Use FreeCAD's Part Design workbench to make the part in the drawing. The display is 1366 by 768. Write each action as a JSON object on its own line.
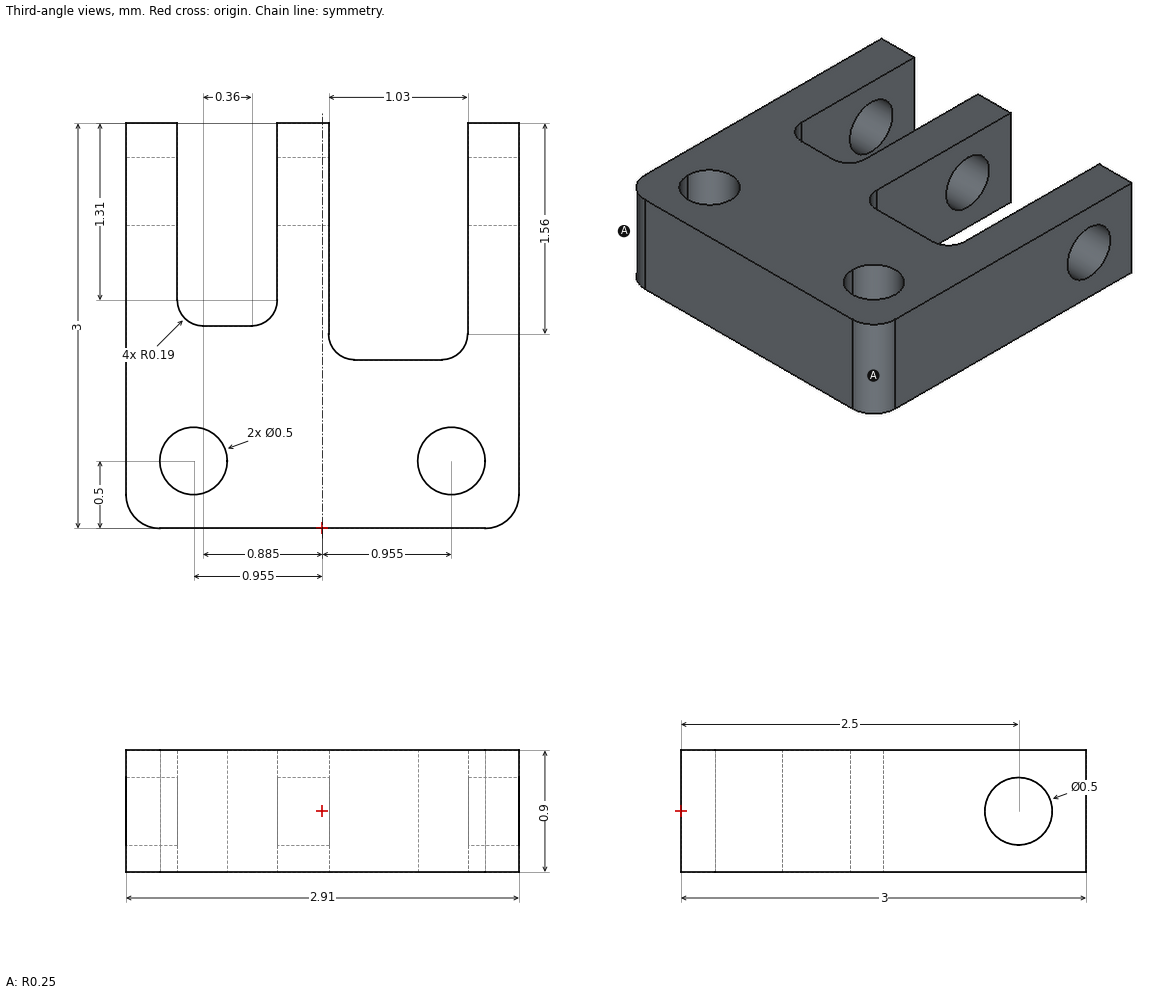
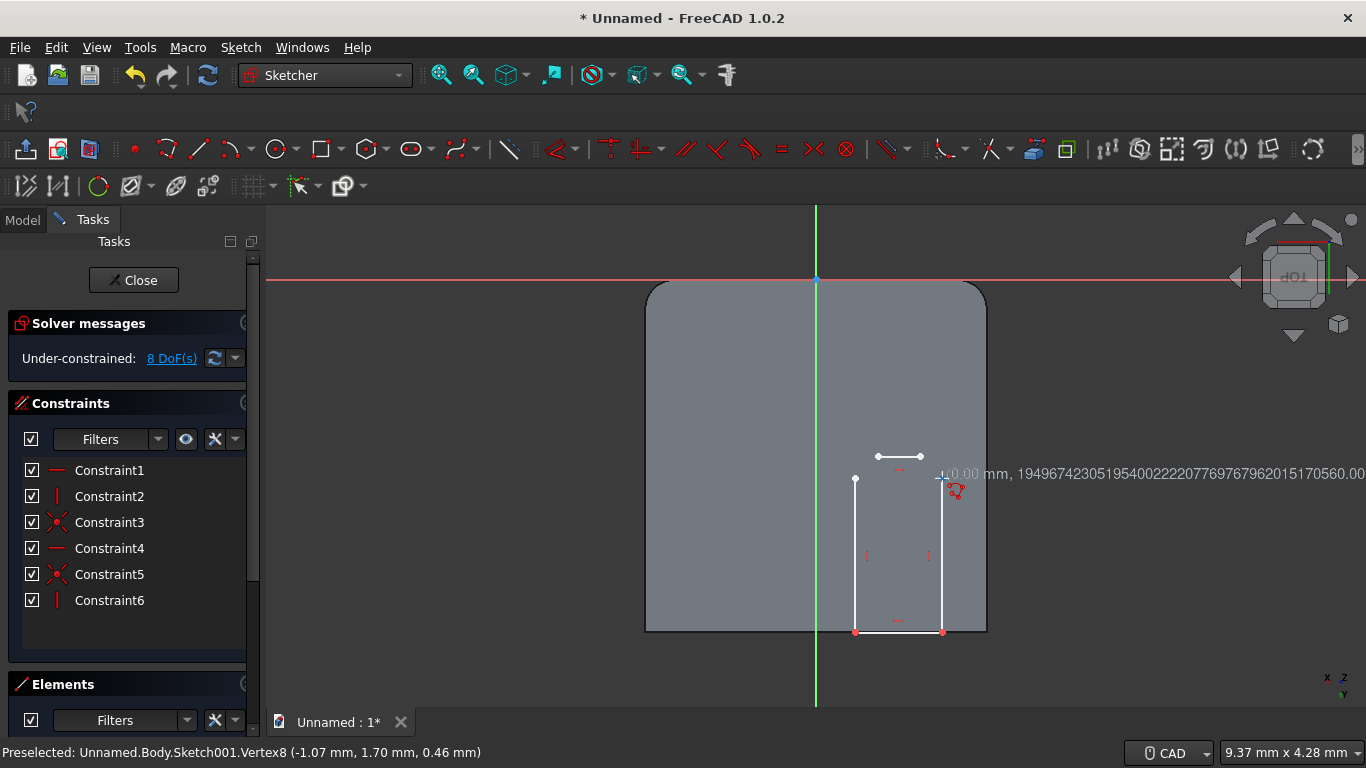
{"action": "key", "text": "g 3 a"}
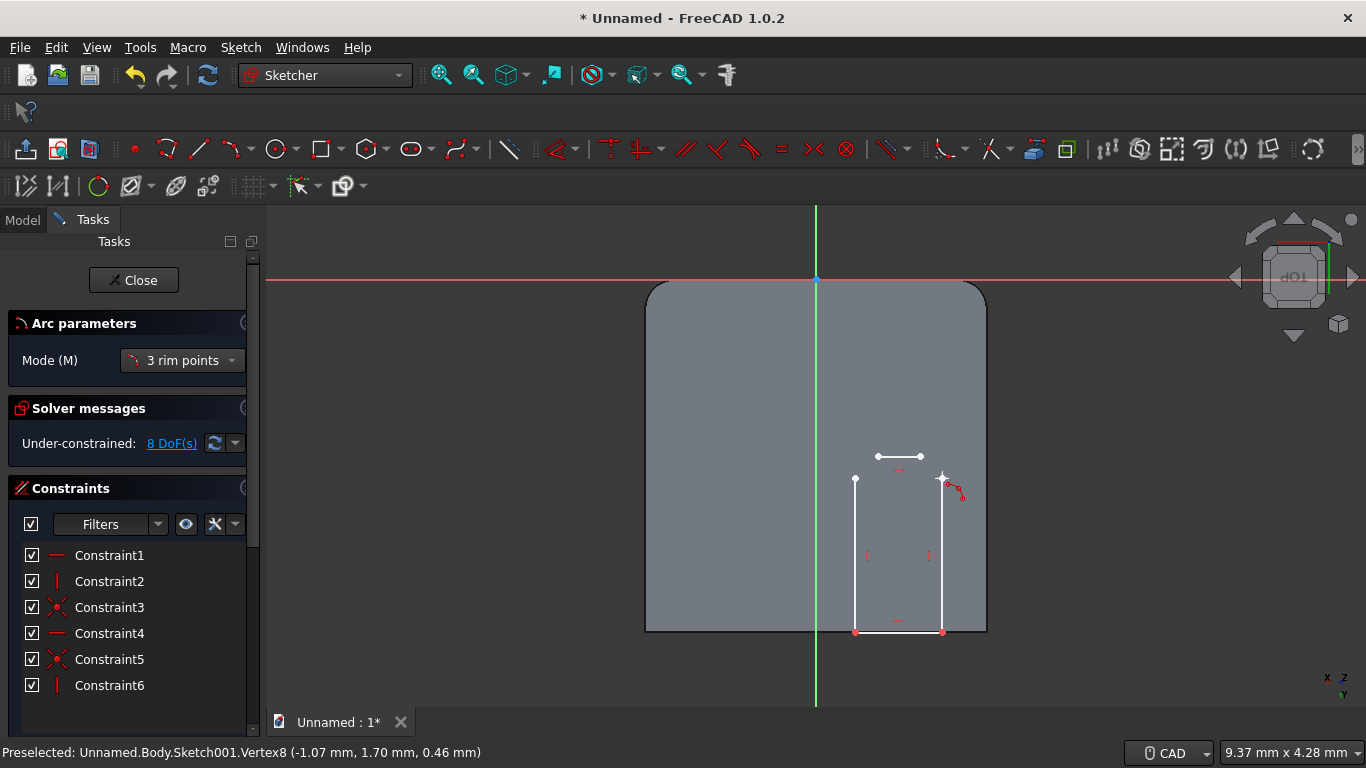
{"action": "left_click", "coordinate": [878, 457]}
{"action": "left_click", "coordinate": [855, 479]}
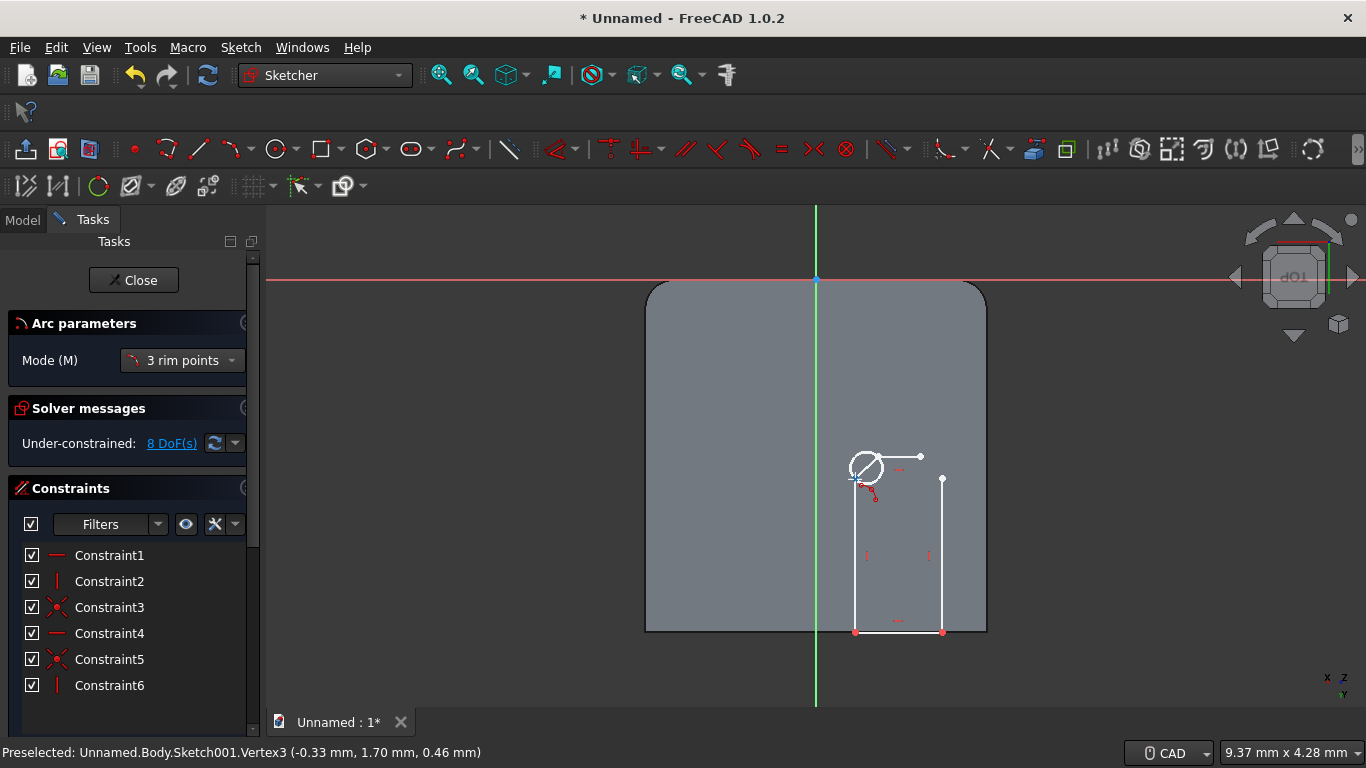
{"action": "scroll", "coordinate": [862, 463], "scroll_direction": "up", "scroll_amount": 5}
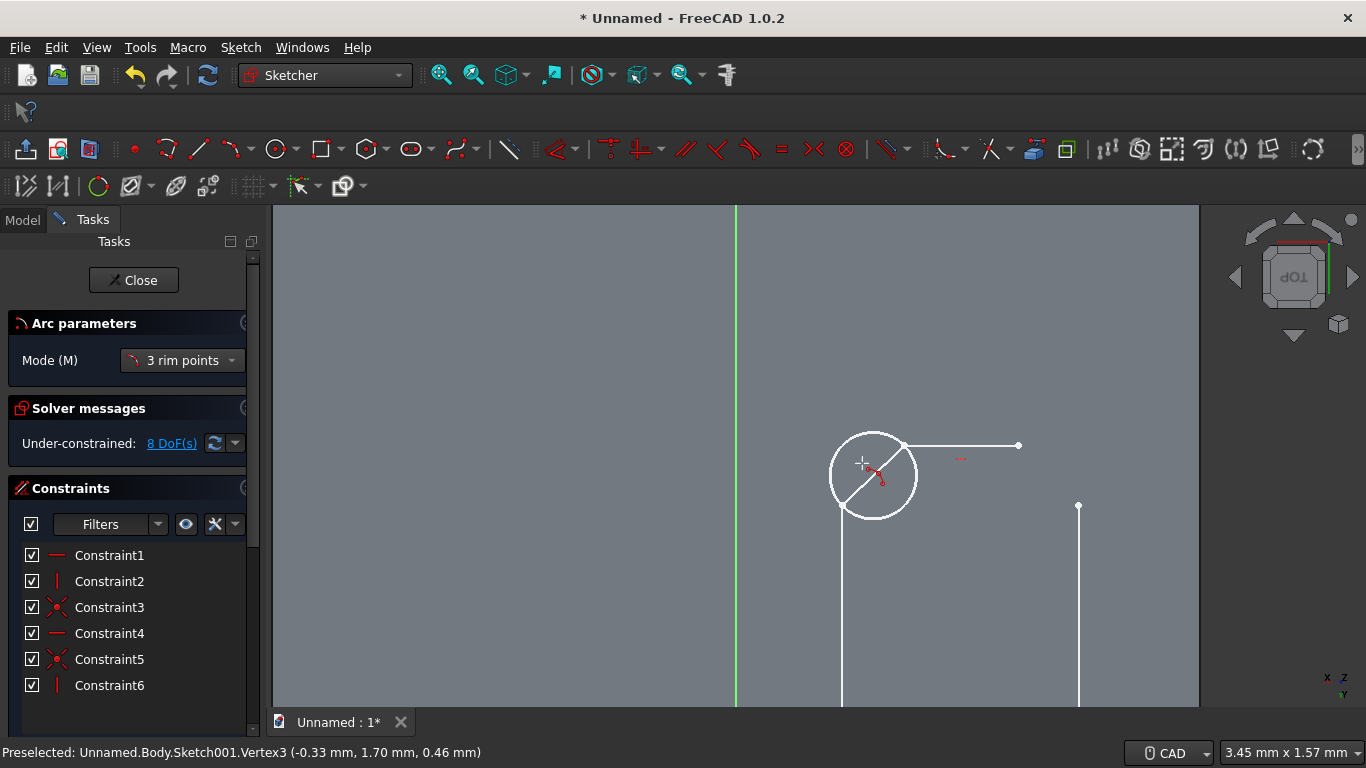
{"action": "left_click", "coordinate": [861, 461]}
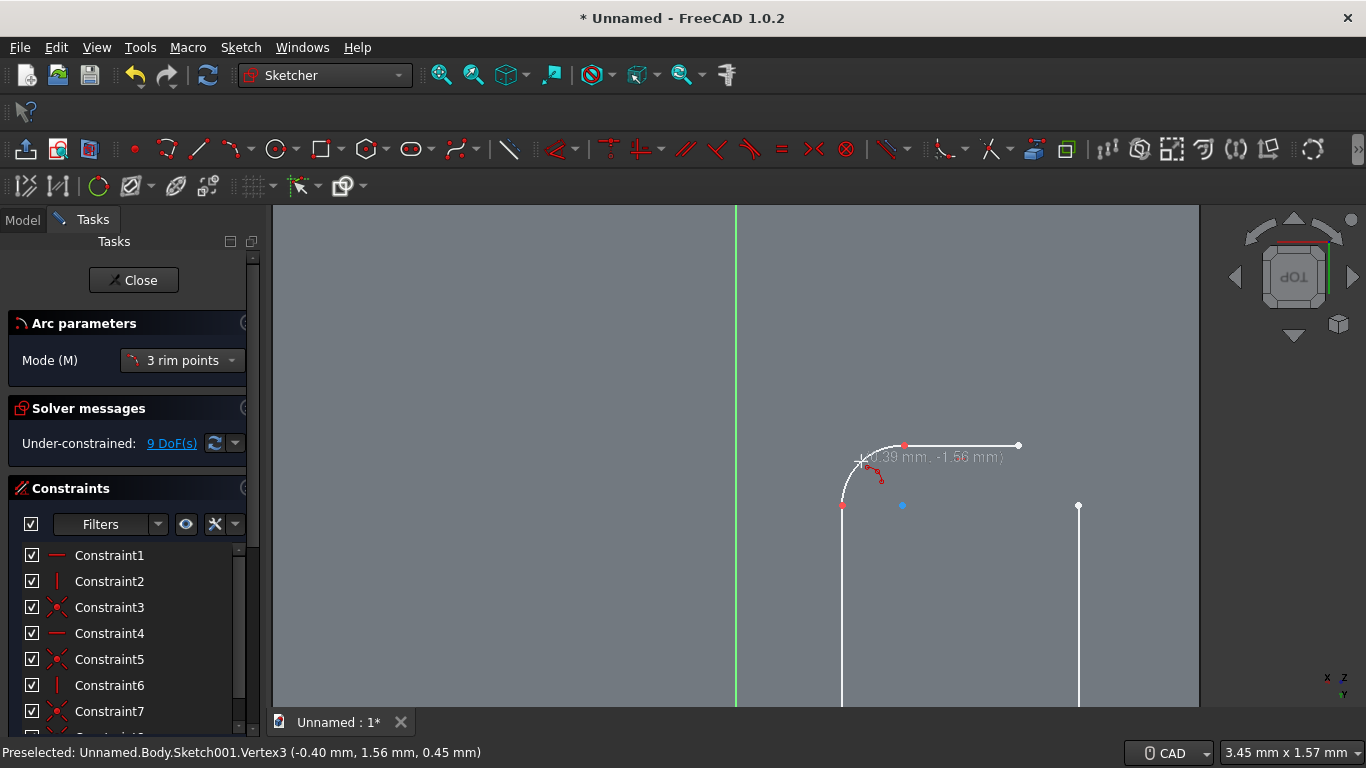
{"action": "left_click", "coordinate": [1079, 506]}
{"action": "left_click", "coordinate": [1019, 446]}
{"action": "left_click", "coordinate": [1061, 461]}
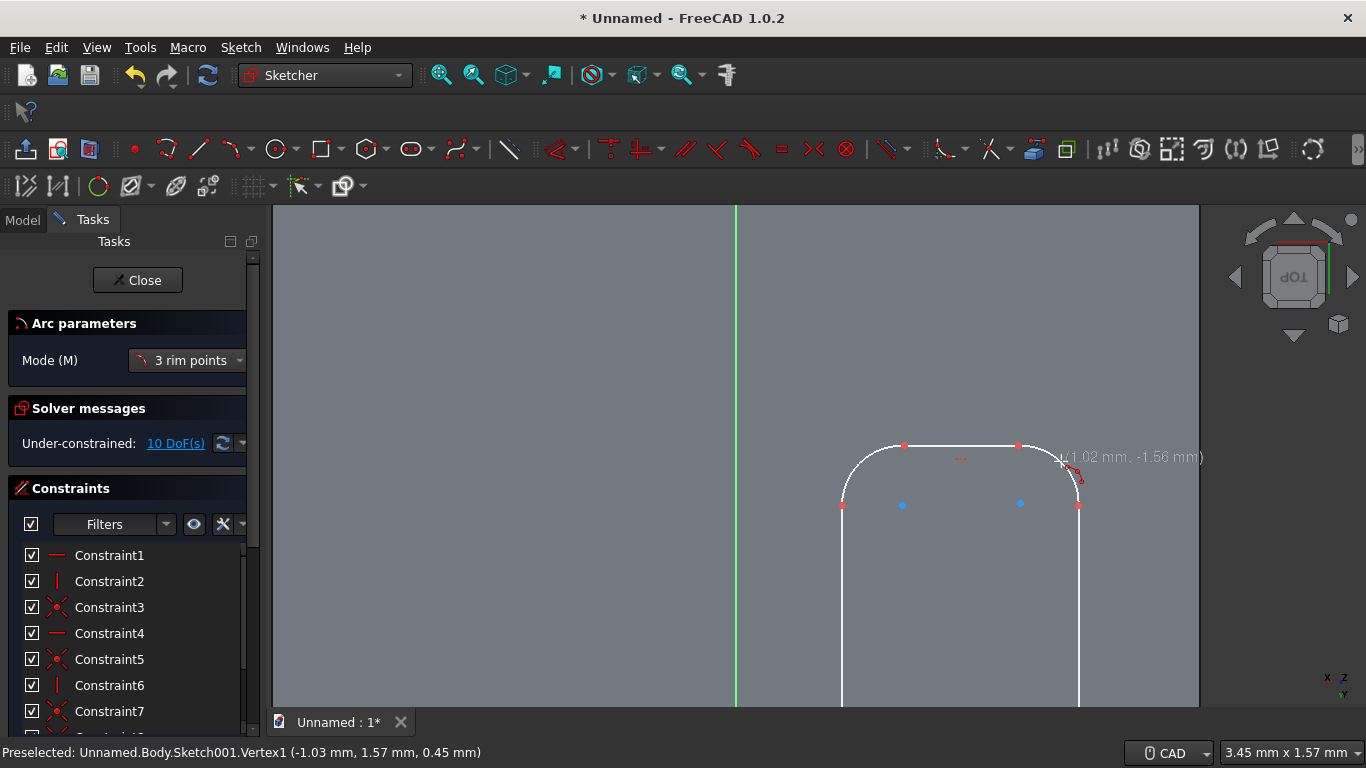
{"action": "left_click", "coordinate": [168, 150]}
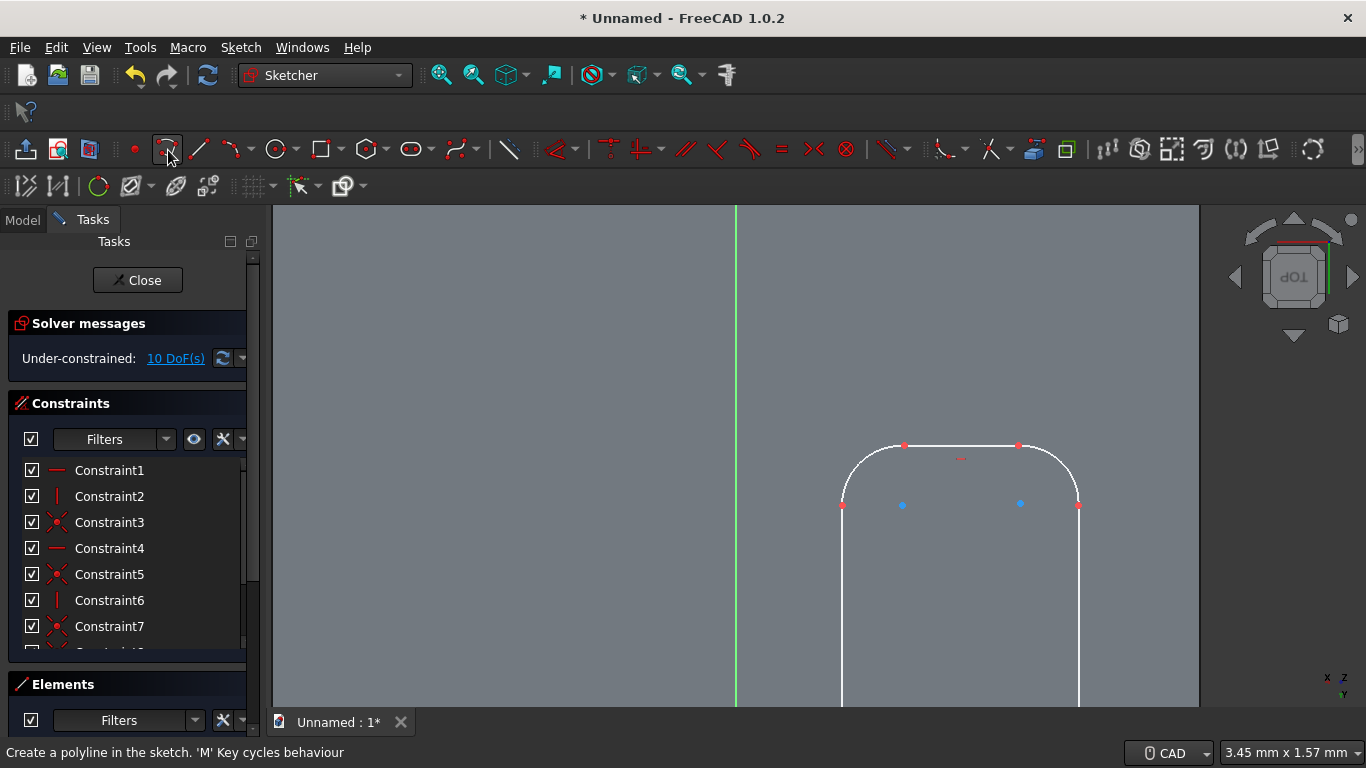
{"action": "left_click", "coordinate": [393, 424]}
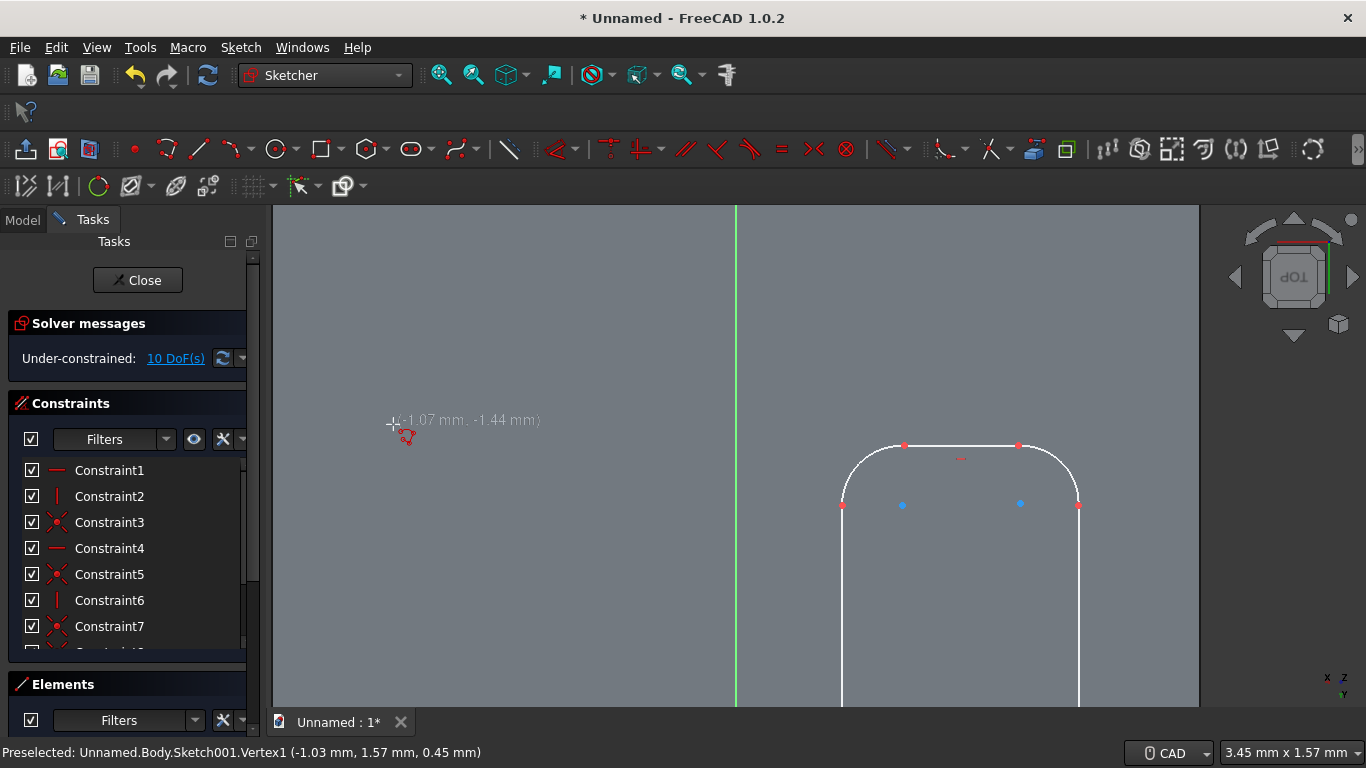
{"action": "scroll", "coordinate": [752, 462], "scroll_direction": "down", "scroll_amount": 6}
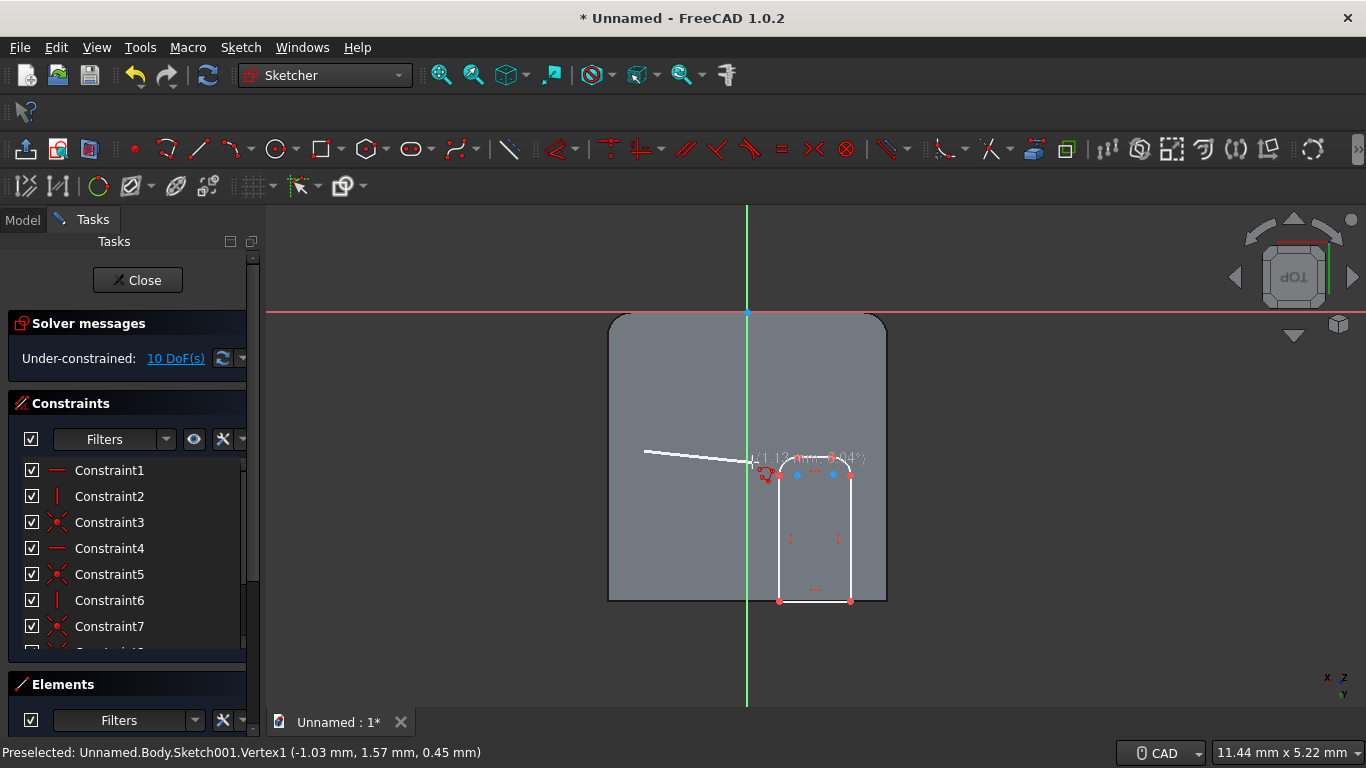
{"action": "left_click", "coordinate": [644, 601]}